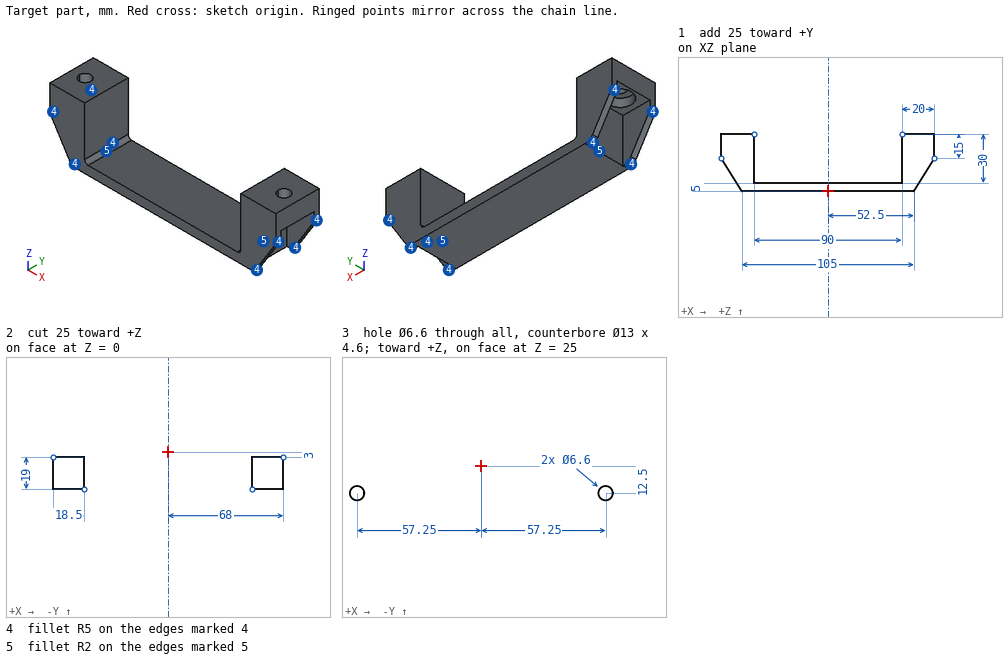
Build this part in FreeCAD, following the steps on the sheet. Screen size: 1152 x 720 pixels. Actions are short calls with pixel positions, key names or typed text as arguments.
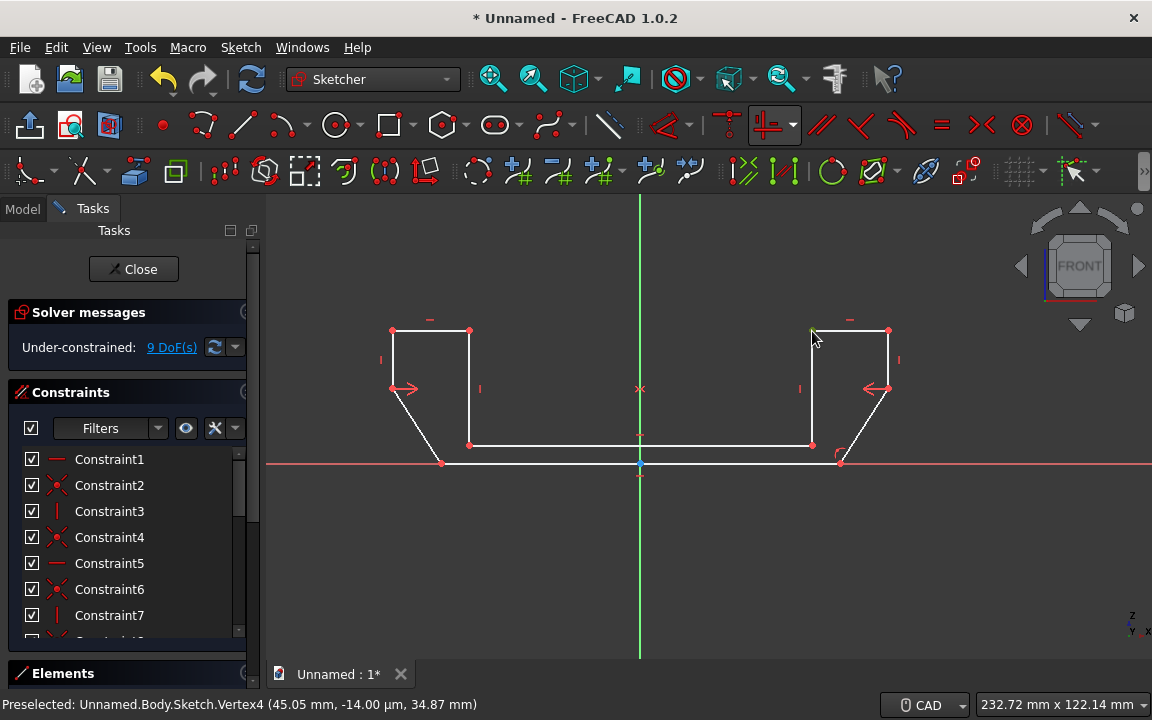
click(469, 331)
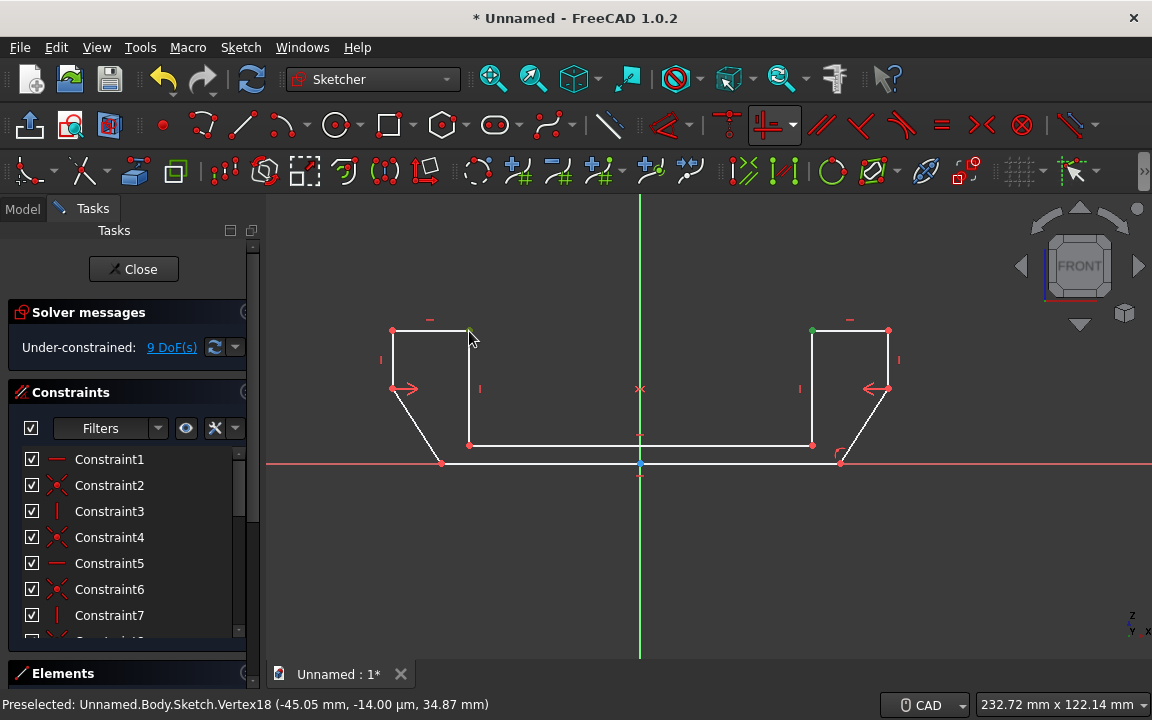
click(640, 602)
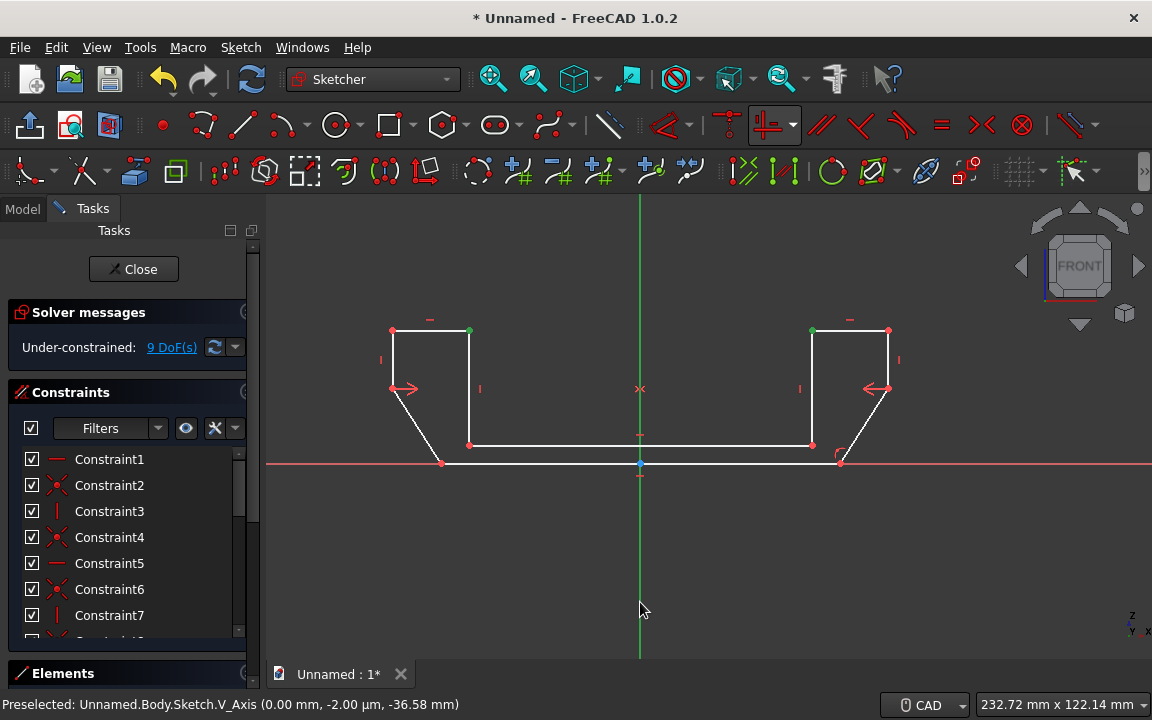
click(982, 126)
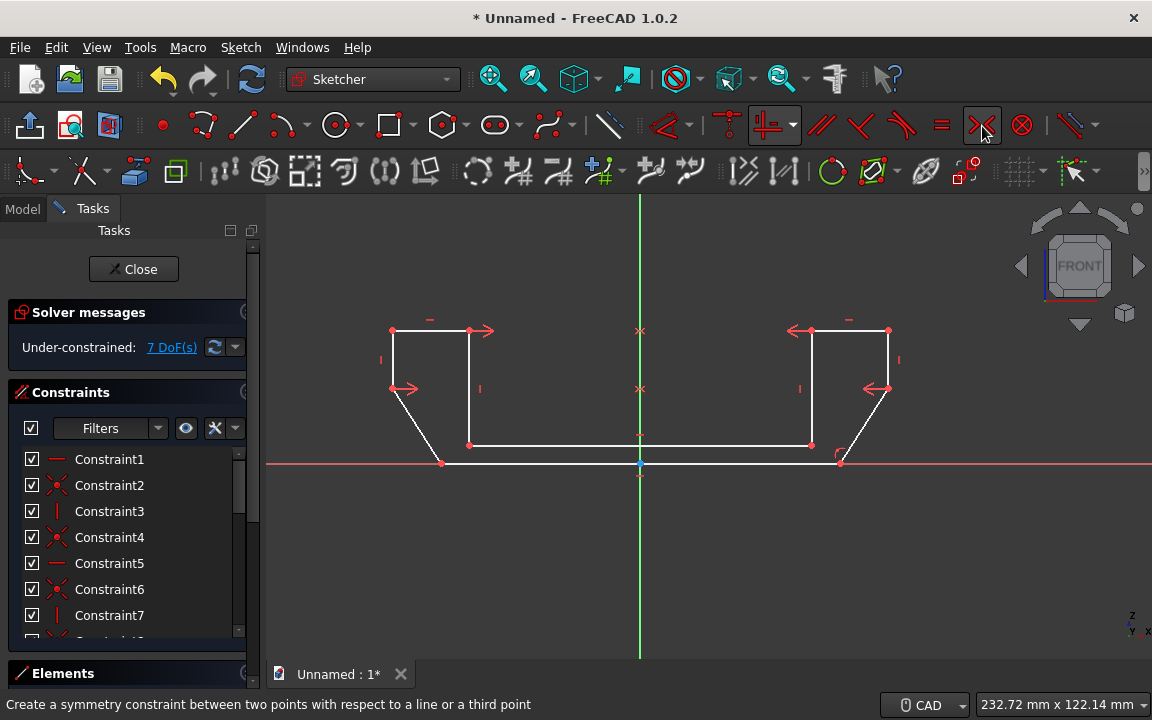
click(572, 446)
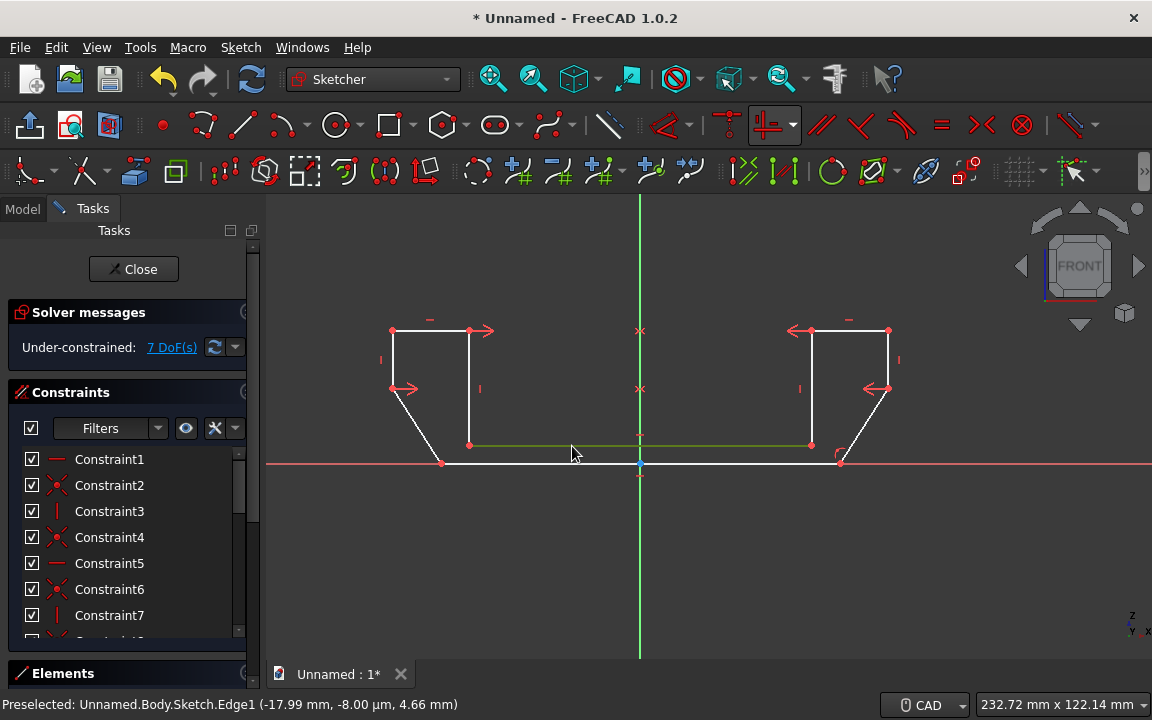
click(692, 126)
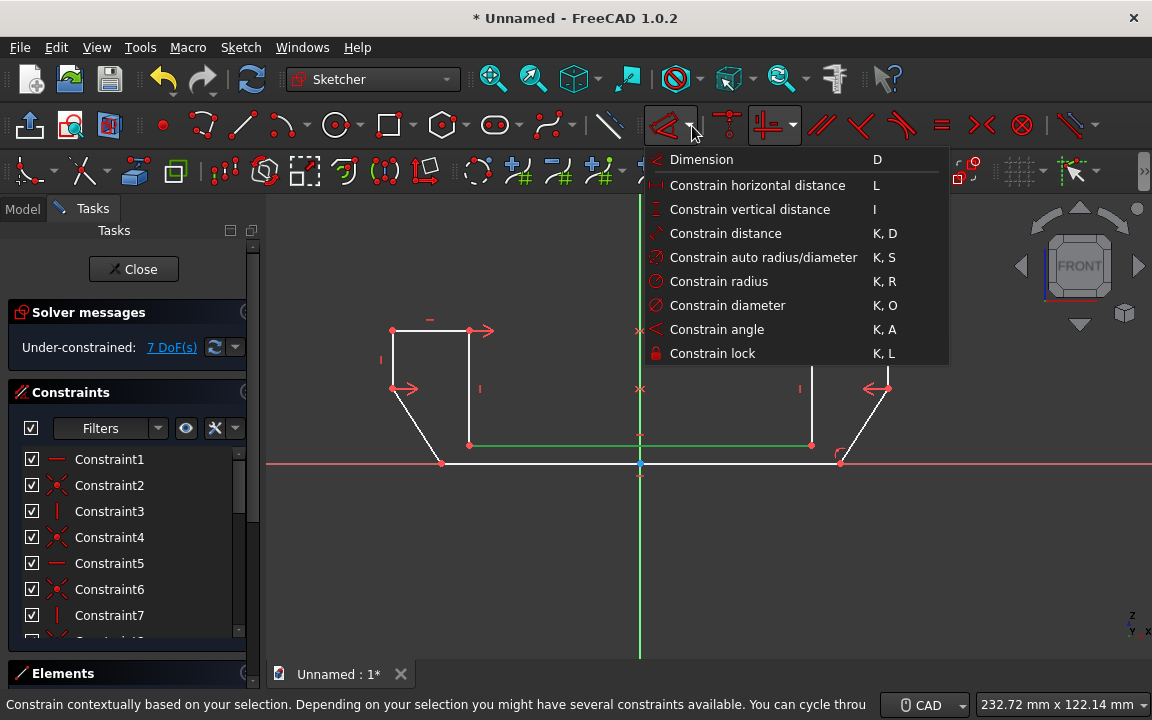
click(797, 185)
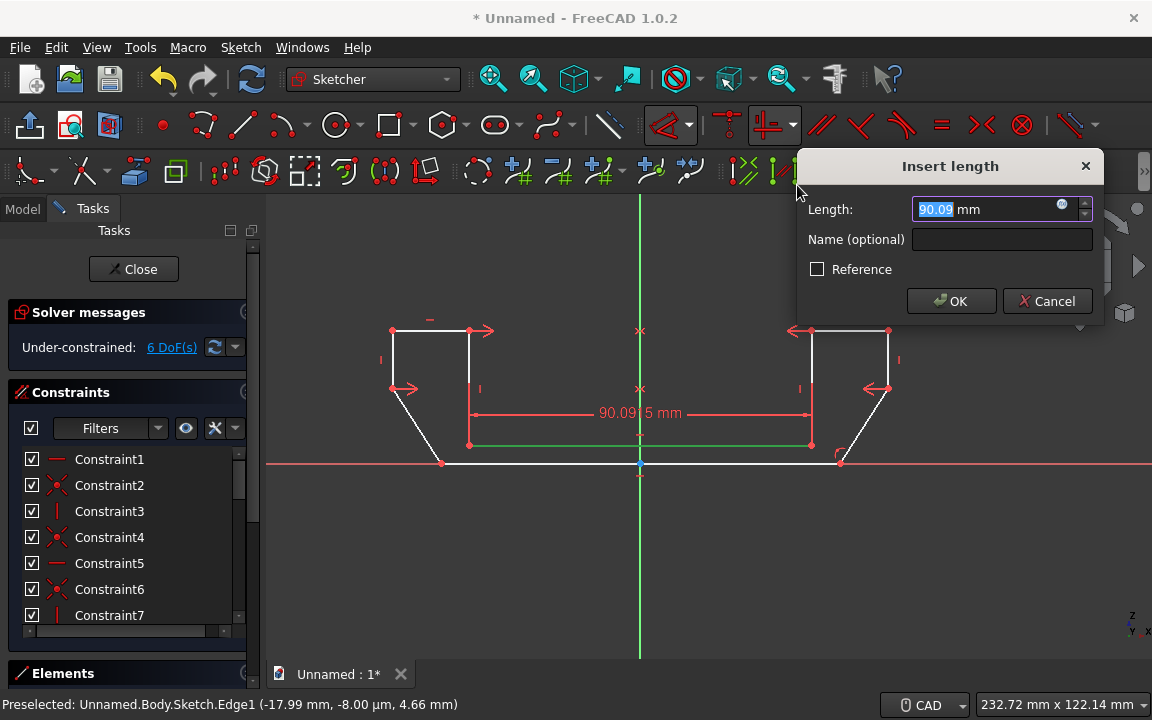
text(90)
key(Return)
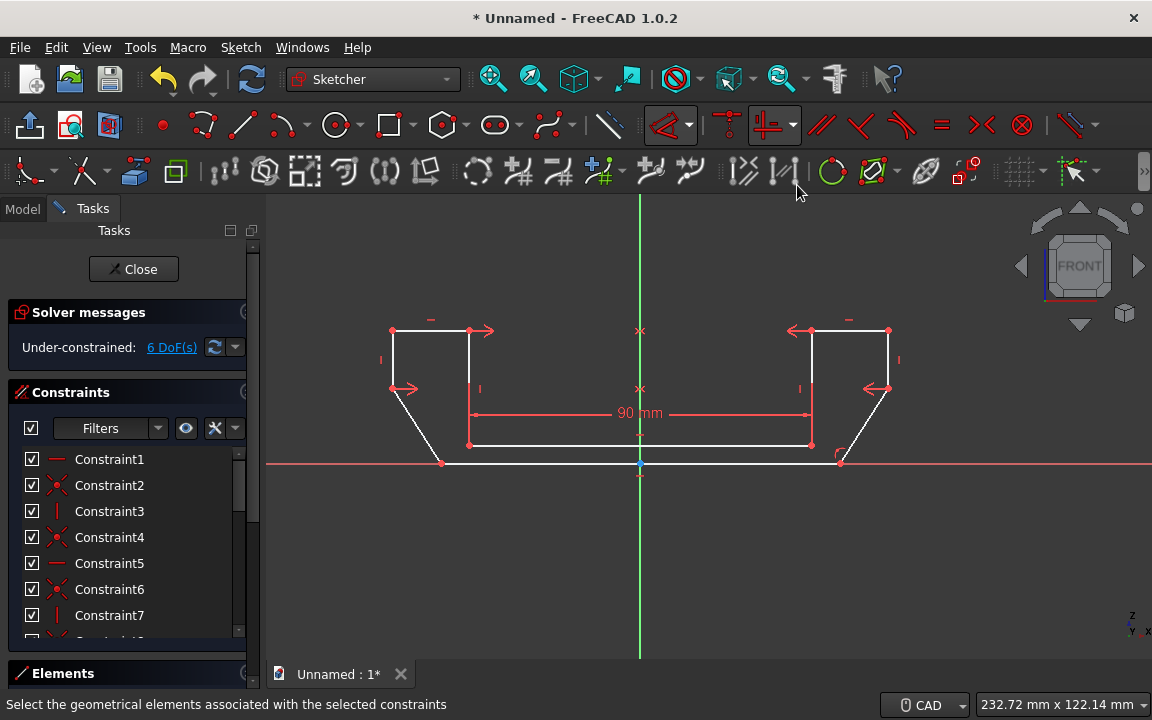
click(812, 411)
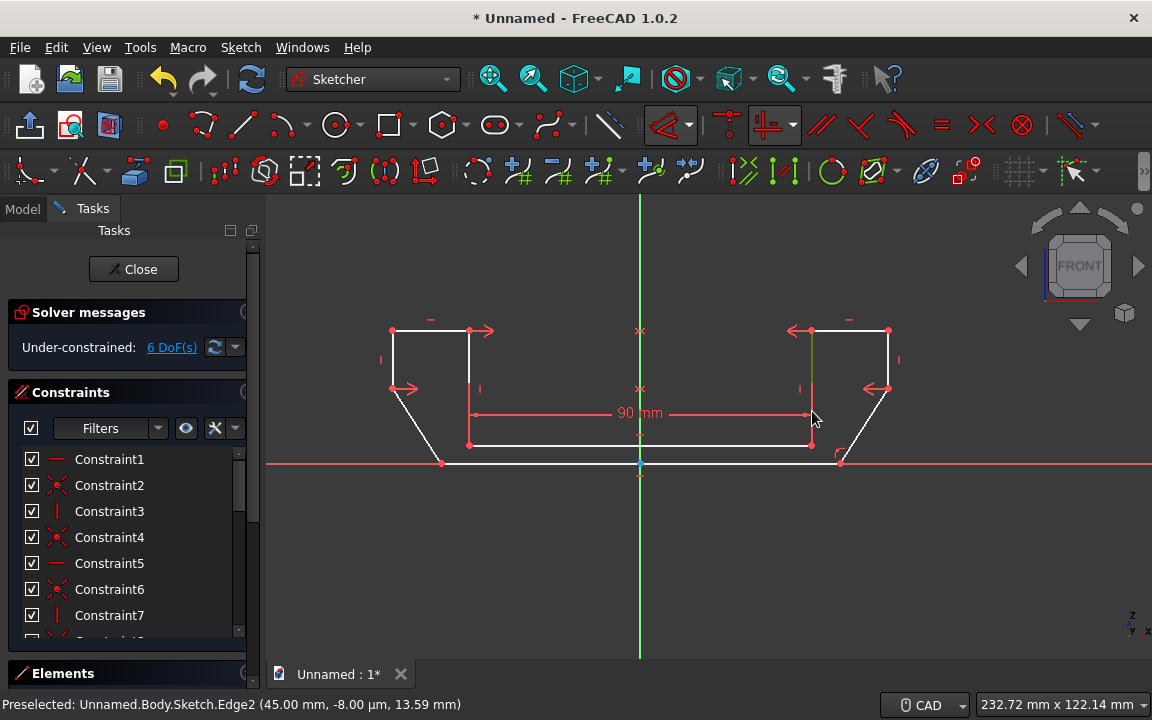
key(i)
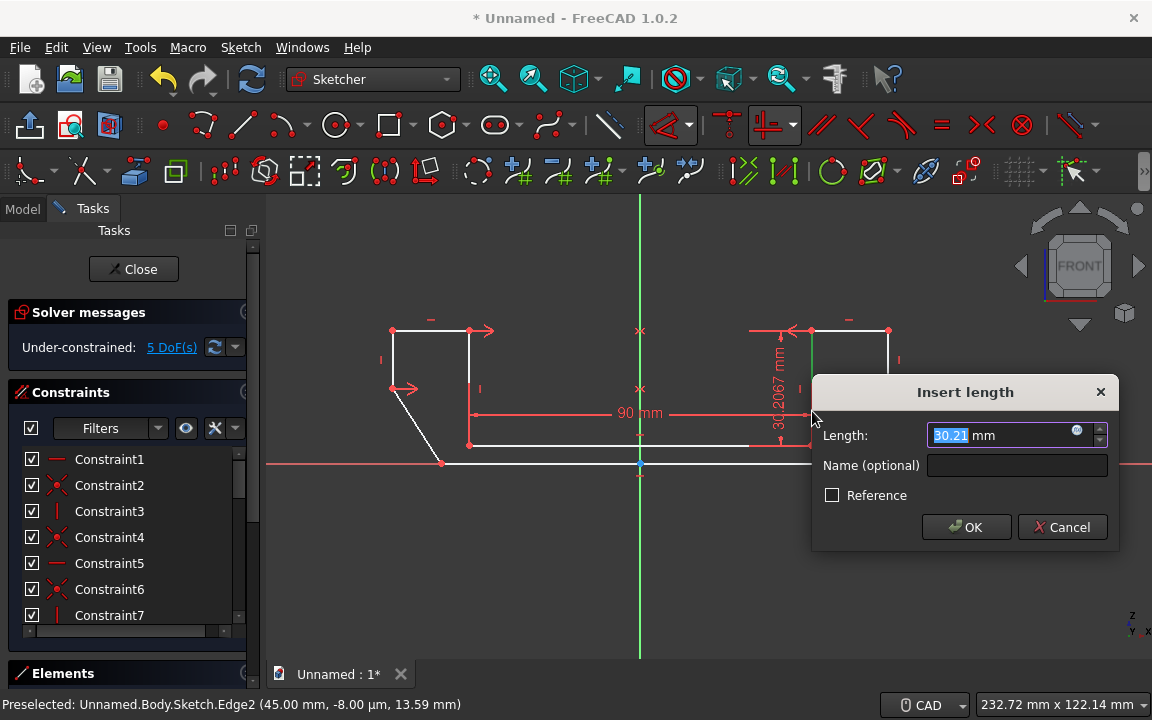
text(30)
key(Return)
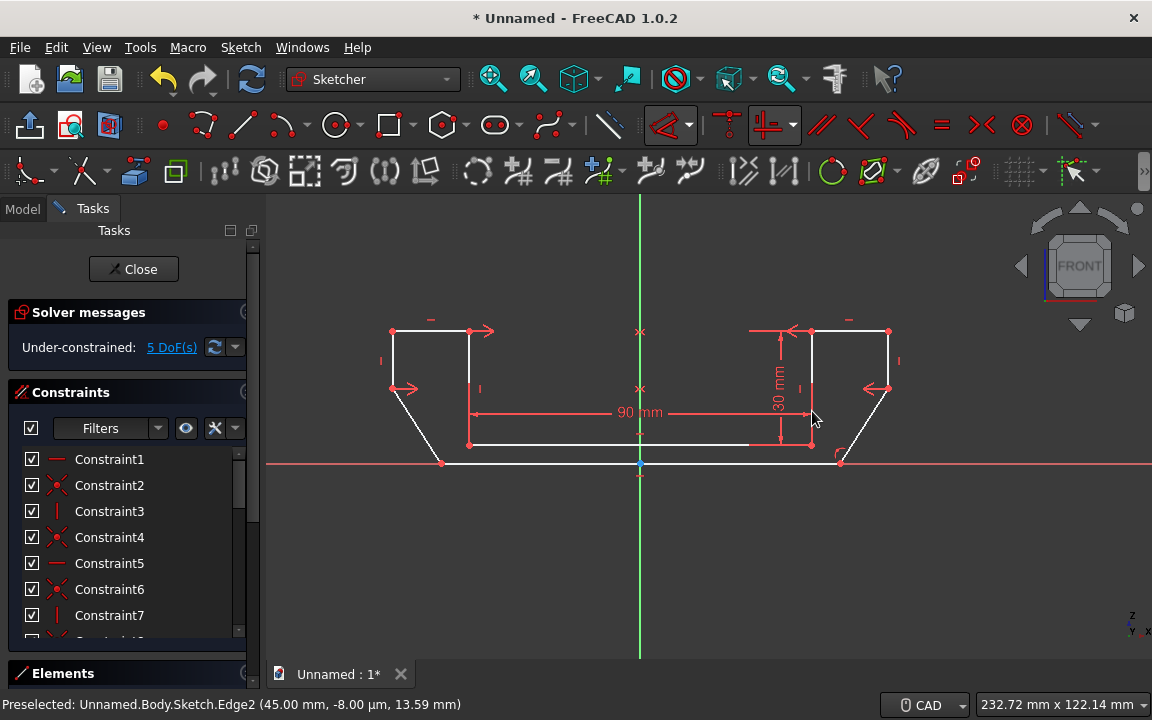
click(835, 331)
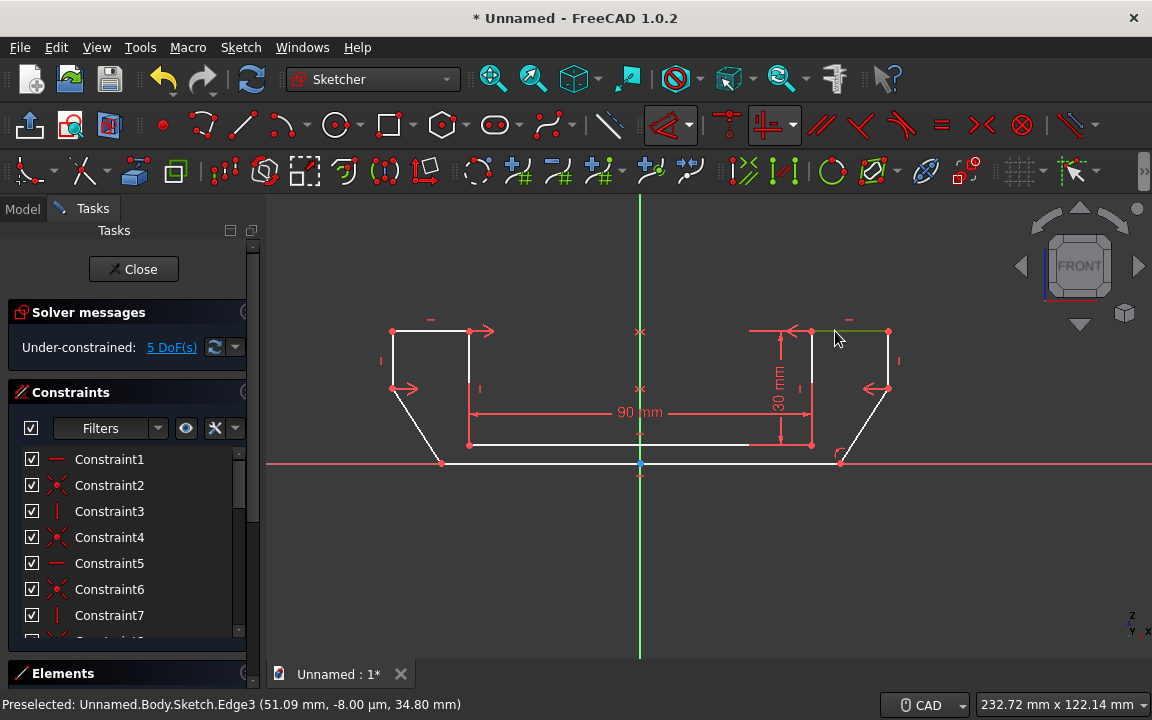
key(l)